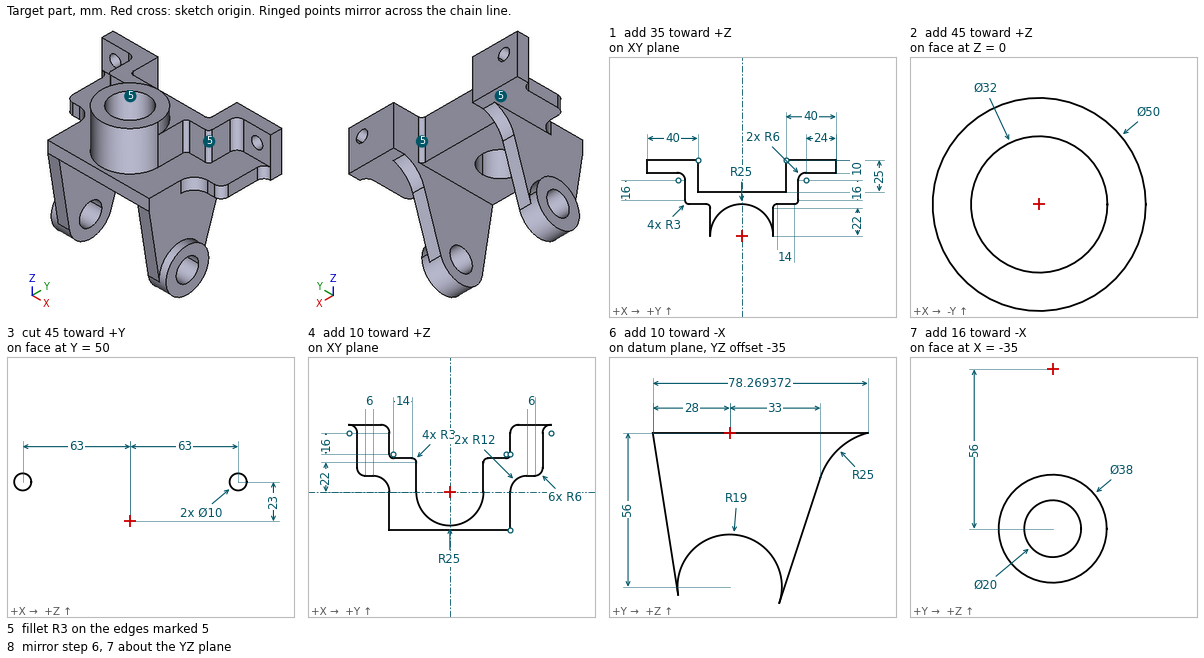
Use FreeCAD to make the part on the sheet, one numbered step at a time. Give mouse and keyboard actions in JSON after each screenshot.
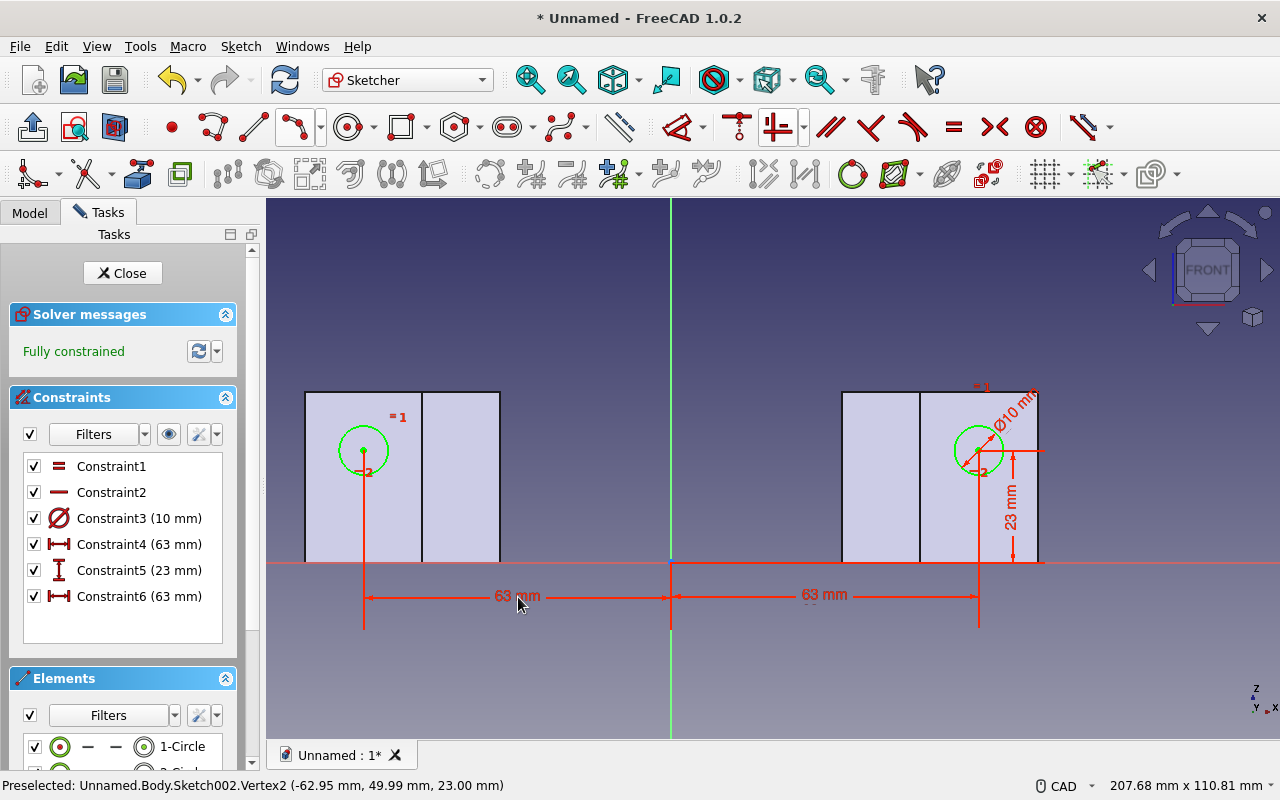
{"action": "left_click", "coordinate": [123, 273]}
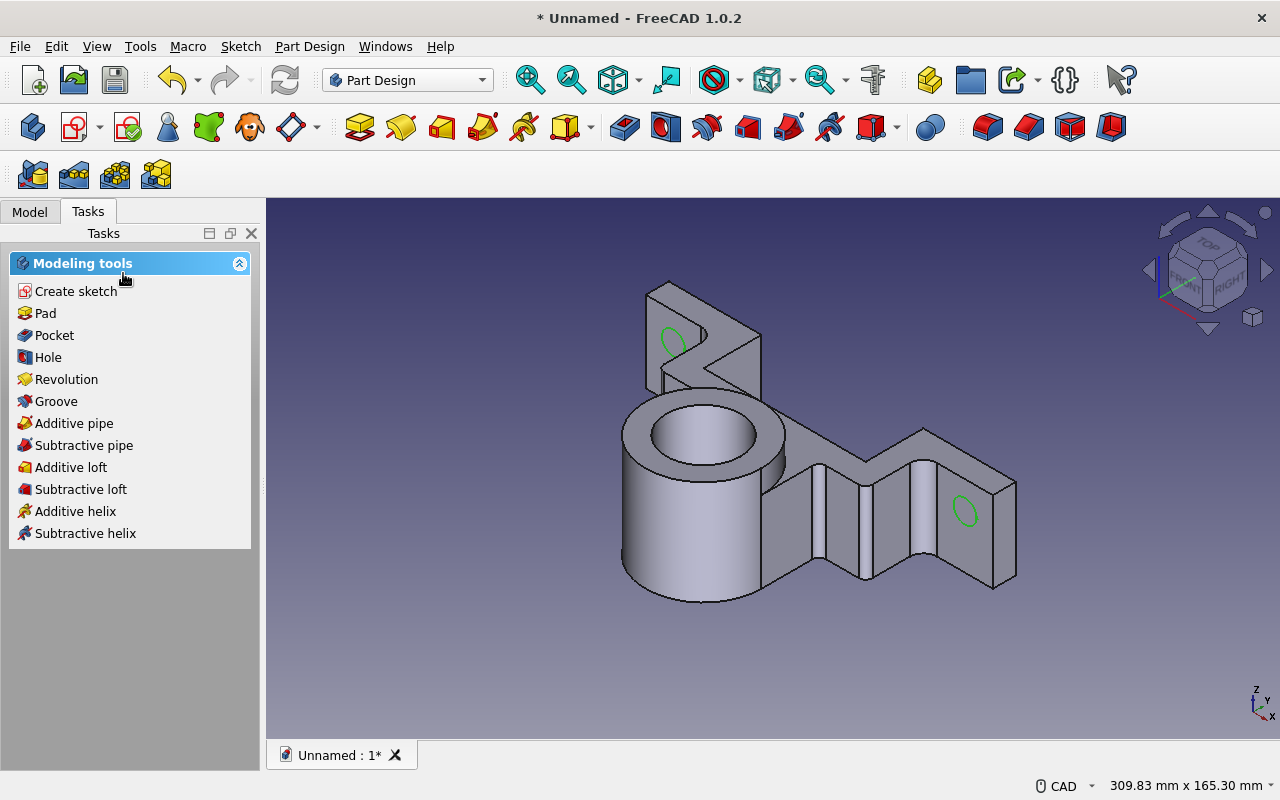
{"action": "left_click", "coordinate": [625, 128]}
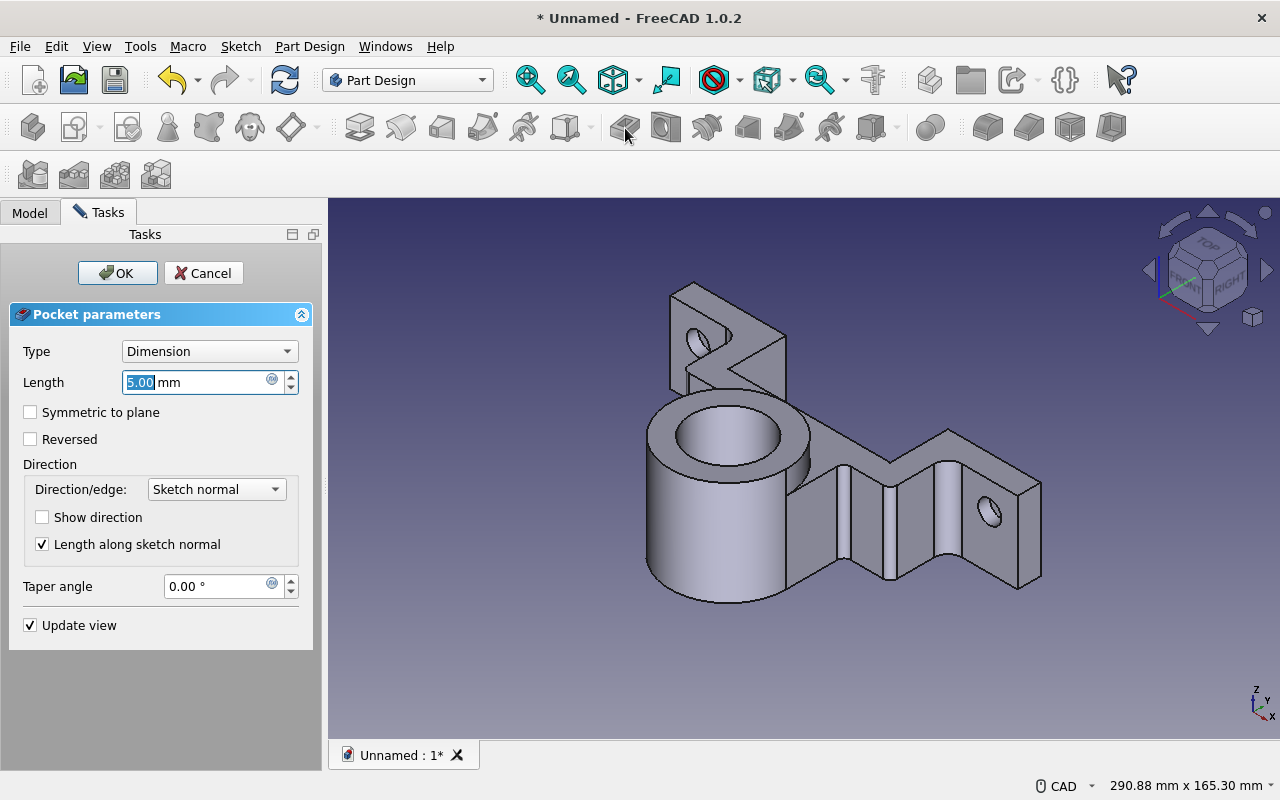
{"action": "type", "text": "45"}
{"action": "key", "text": "Tab"}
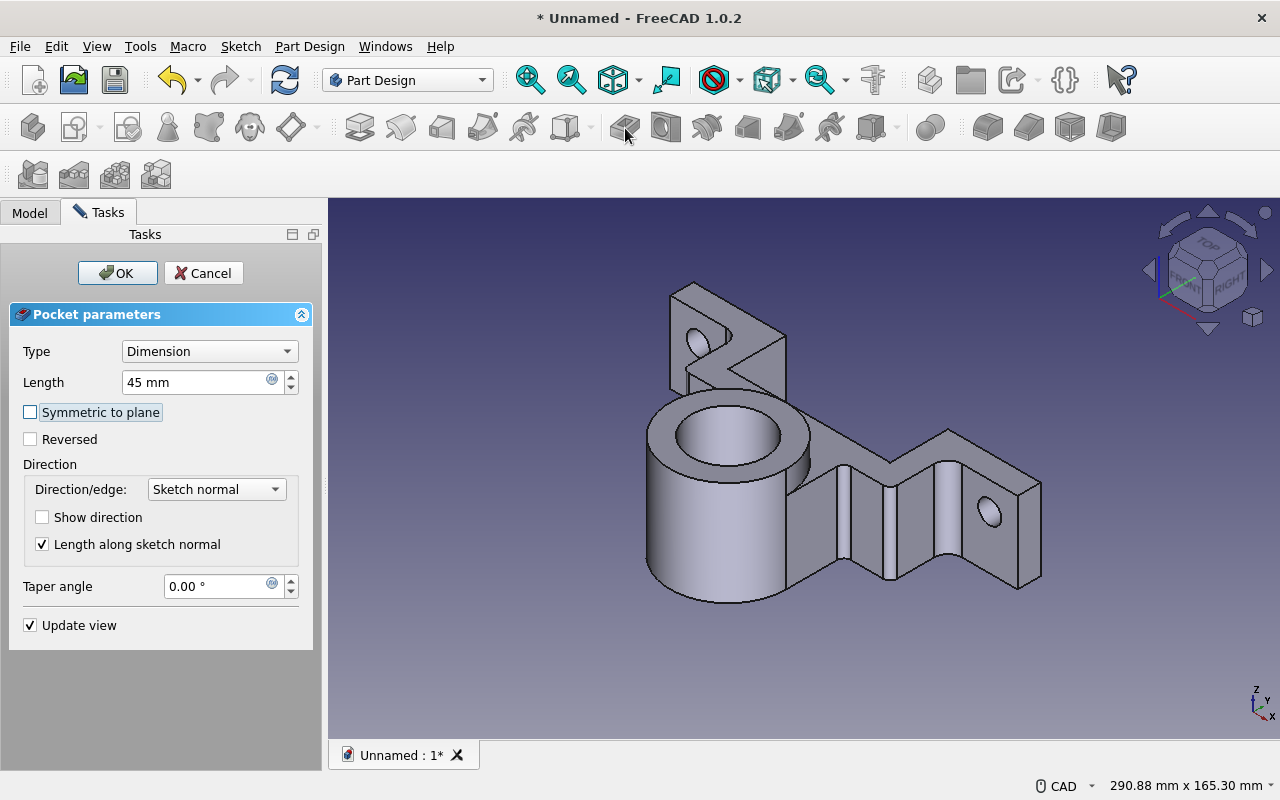
{"action": "left_click", "coordinate": [118, 273]}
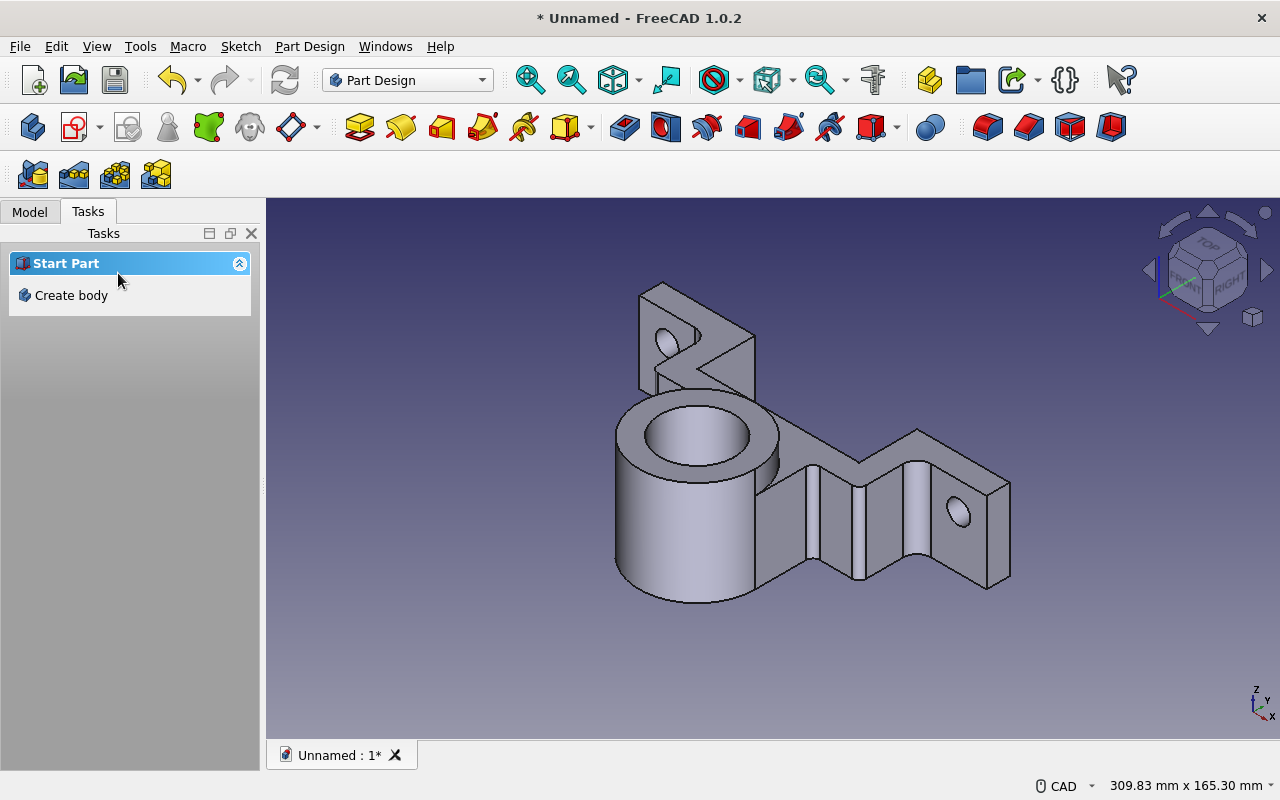
{"action": "left_click", "coordinate": [74, 128]}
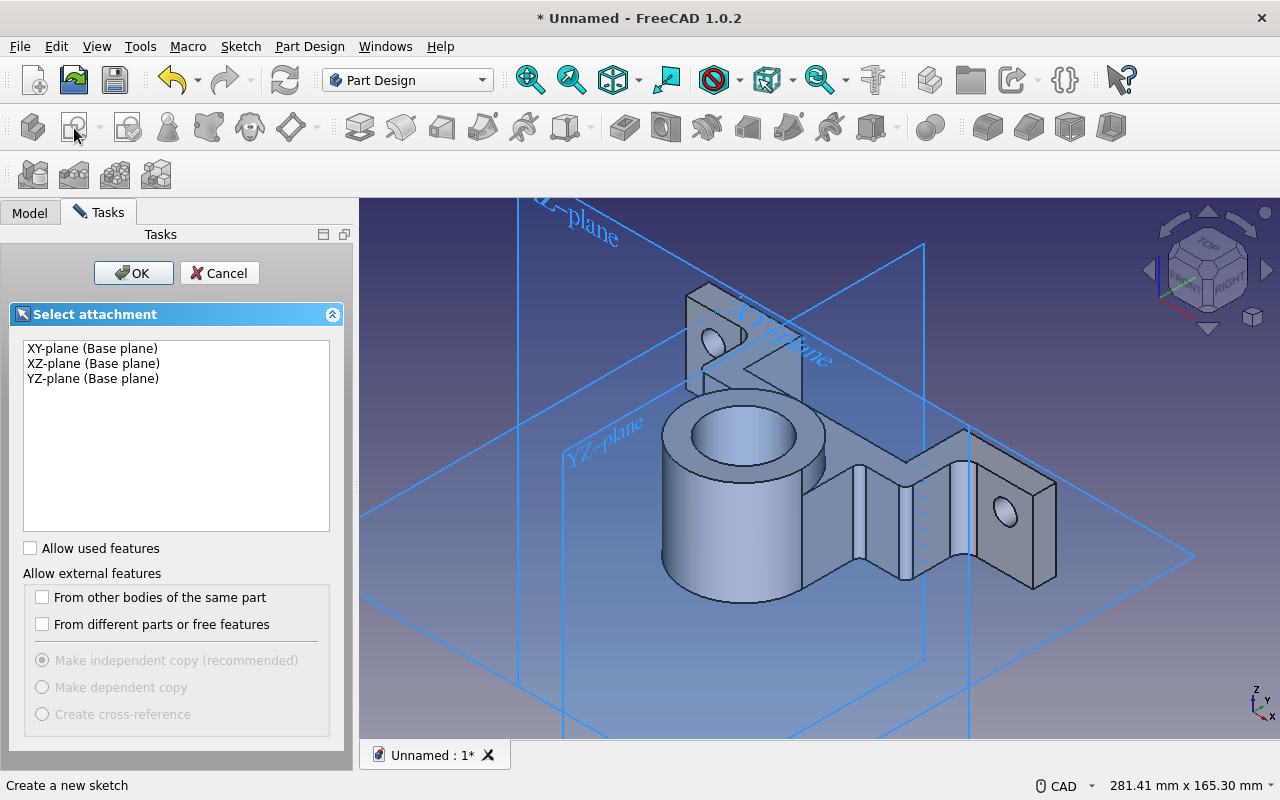
{"action": "left_click", "coordinate": [84, 348]}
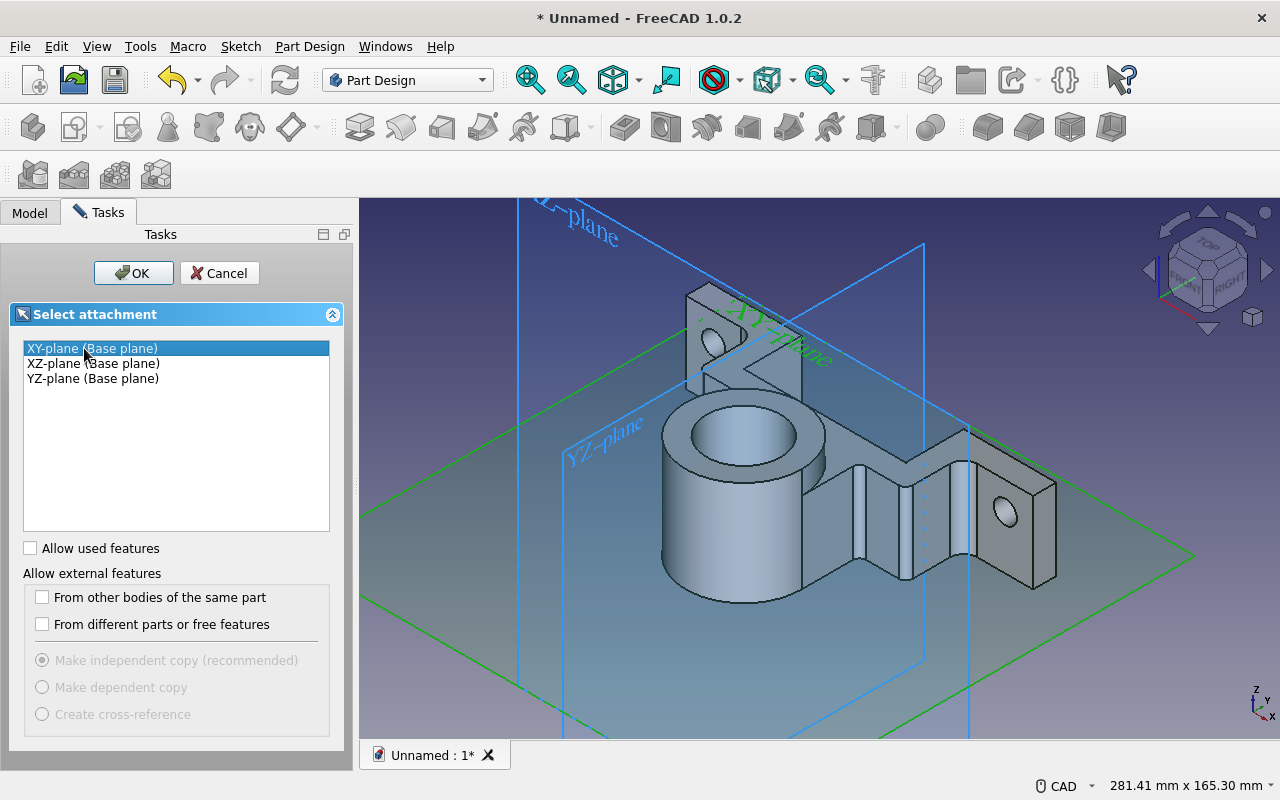
{"action": "left_click", "coordinate": [134, 273]}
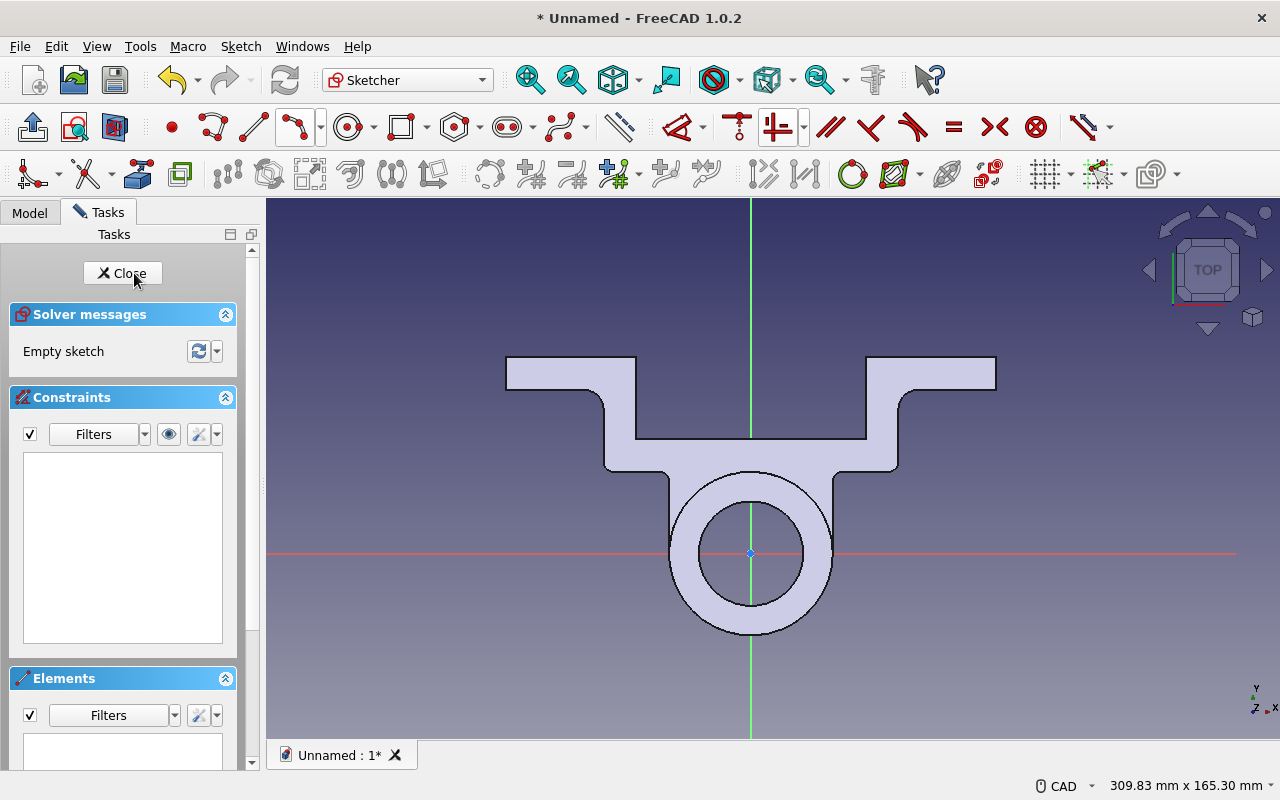
{"action": "left_click", "coordinate": [115, 128]}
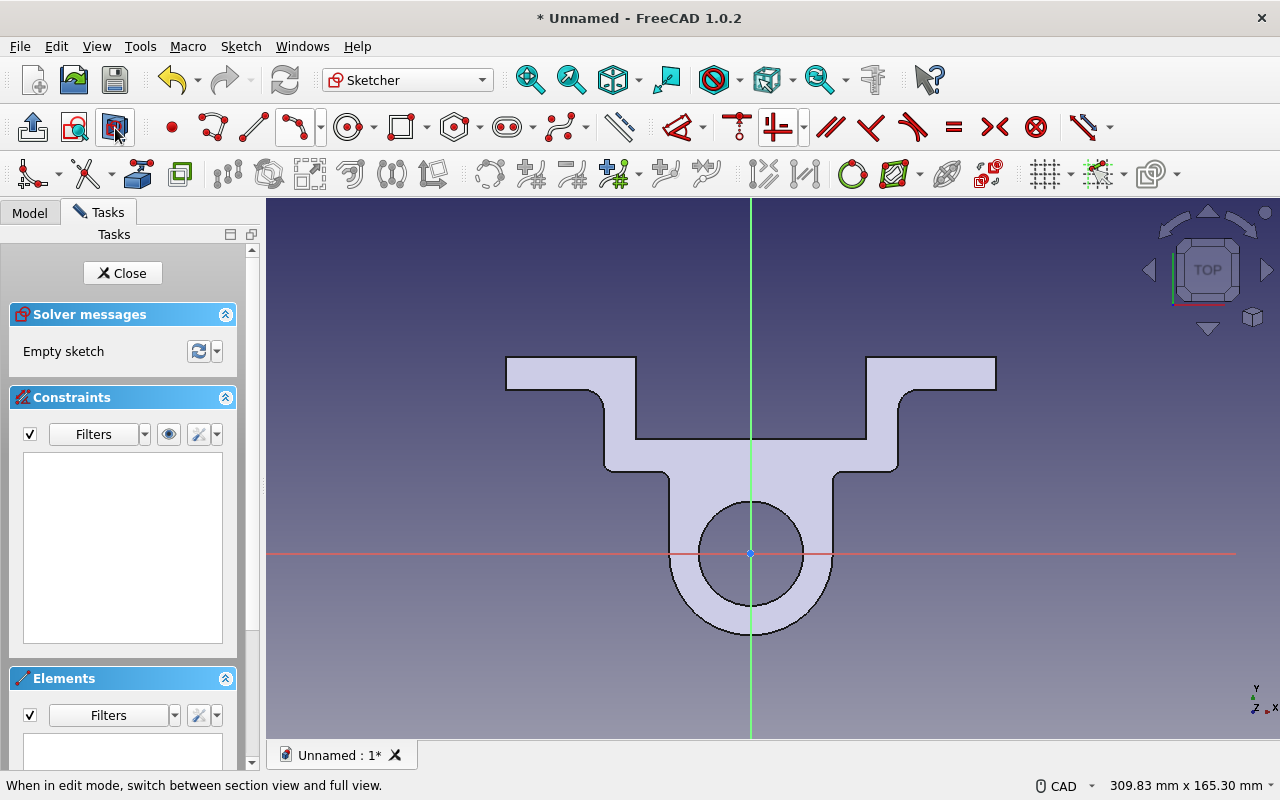
{"action": "left_click", "coordinate": [254, 128]}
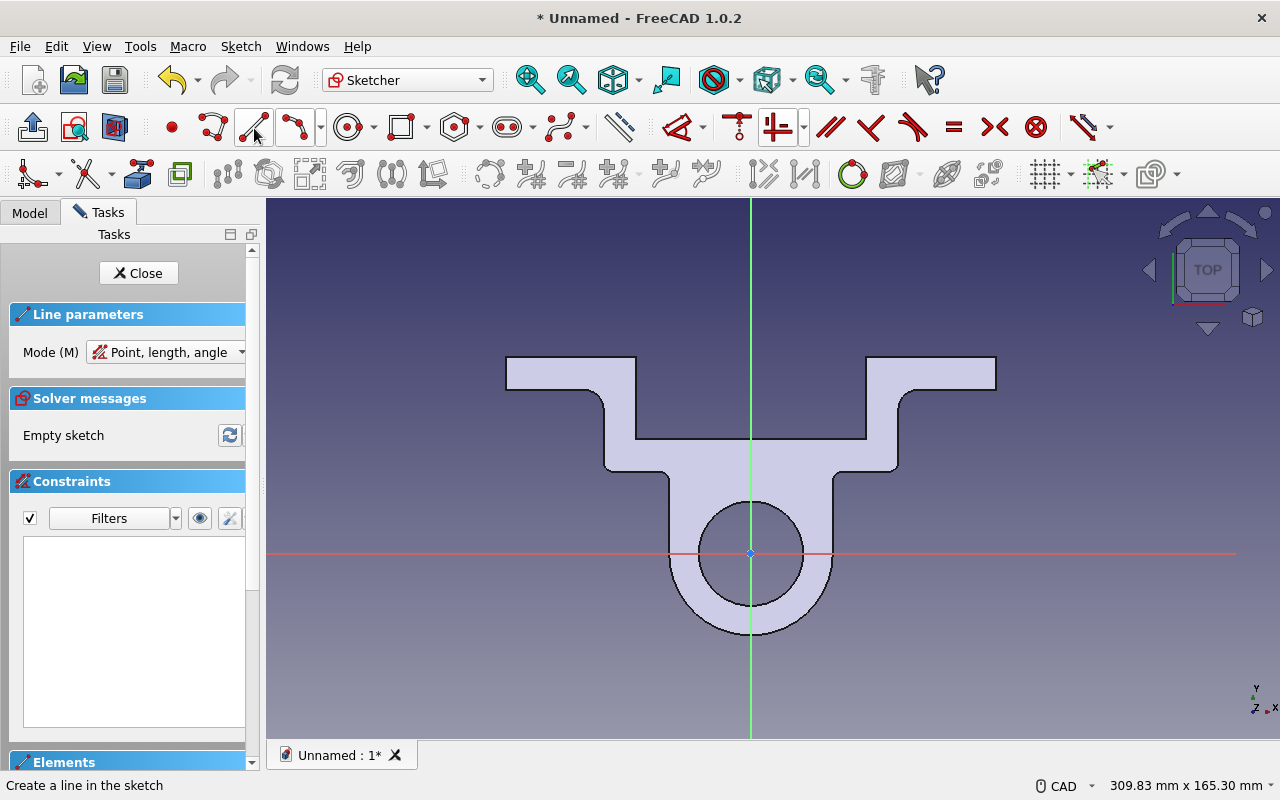
{"action": "left_click", "coordinate": [506, 390]}
{"action": "left_click", "coordinate": [584, 390]}